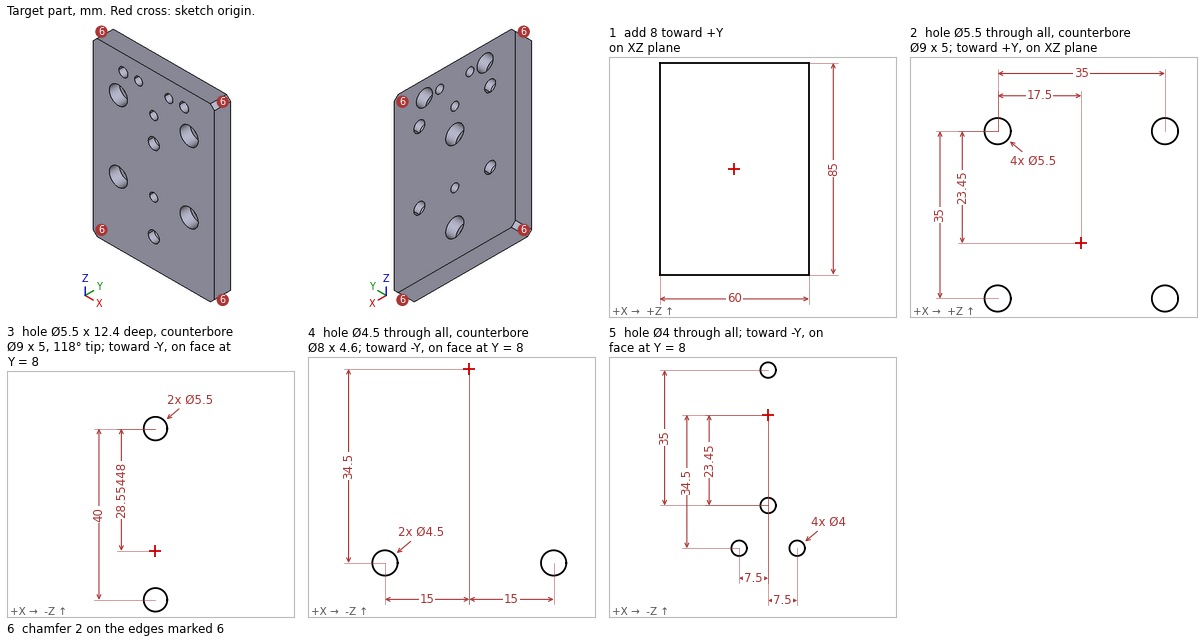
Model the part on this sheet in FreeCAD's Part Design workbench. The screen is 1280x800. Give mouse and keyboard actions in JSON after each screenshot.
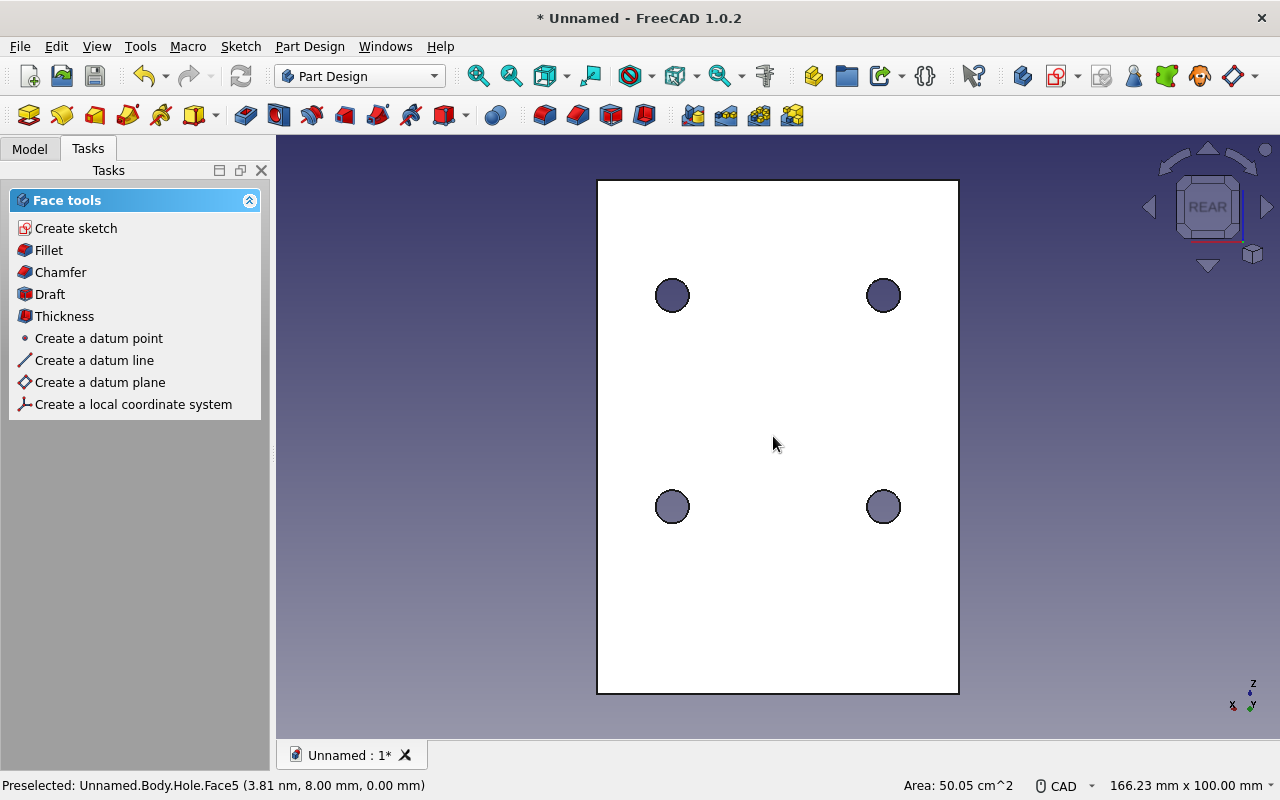
{"action": "left_click", "coordinate": [1056, 76]}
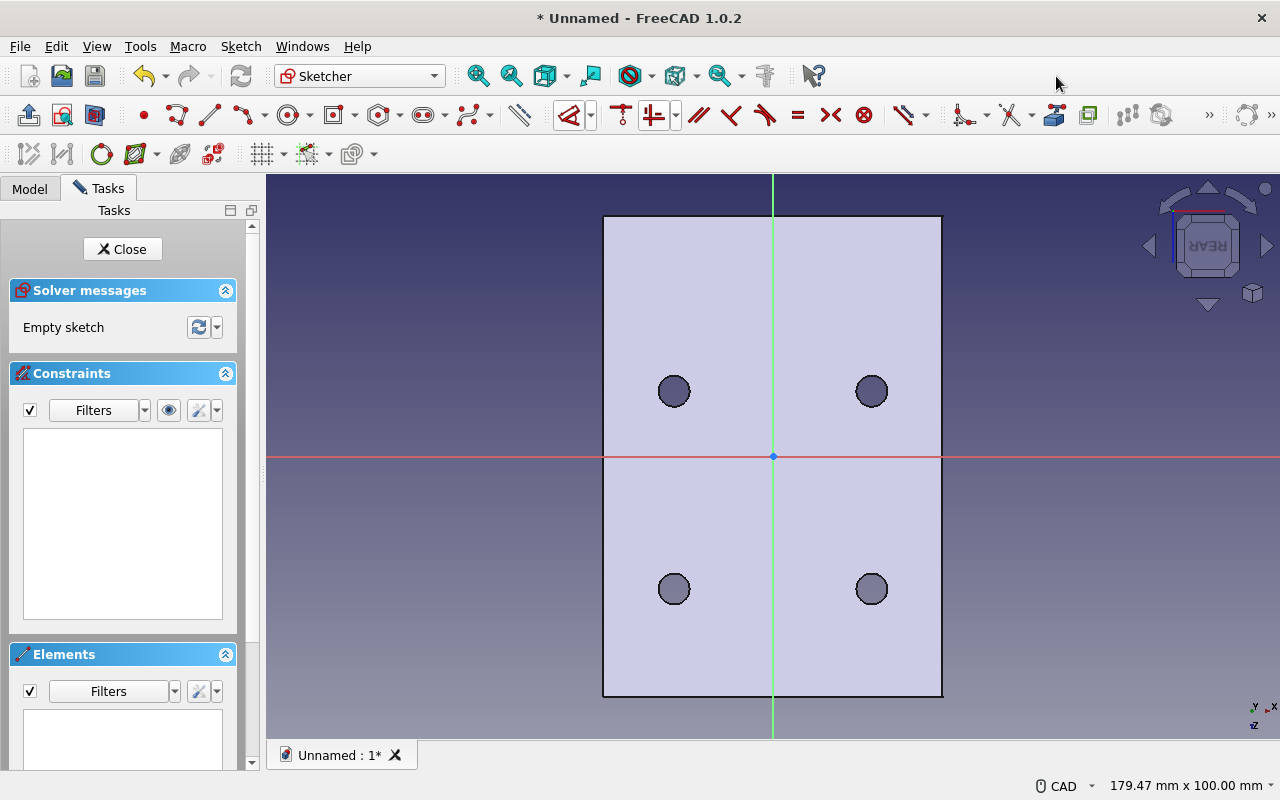
{"action": "scroll", "coordinate": [912, 310], "scroll_direction": "up", "scroll_amount": 2}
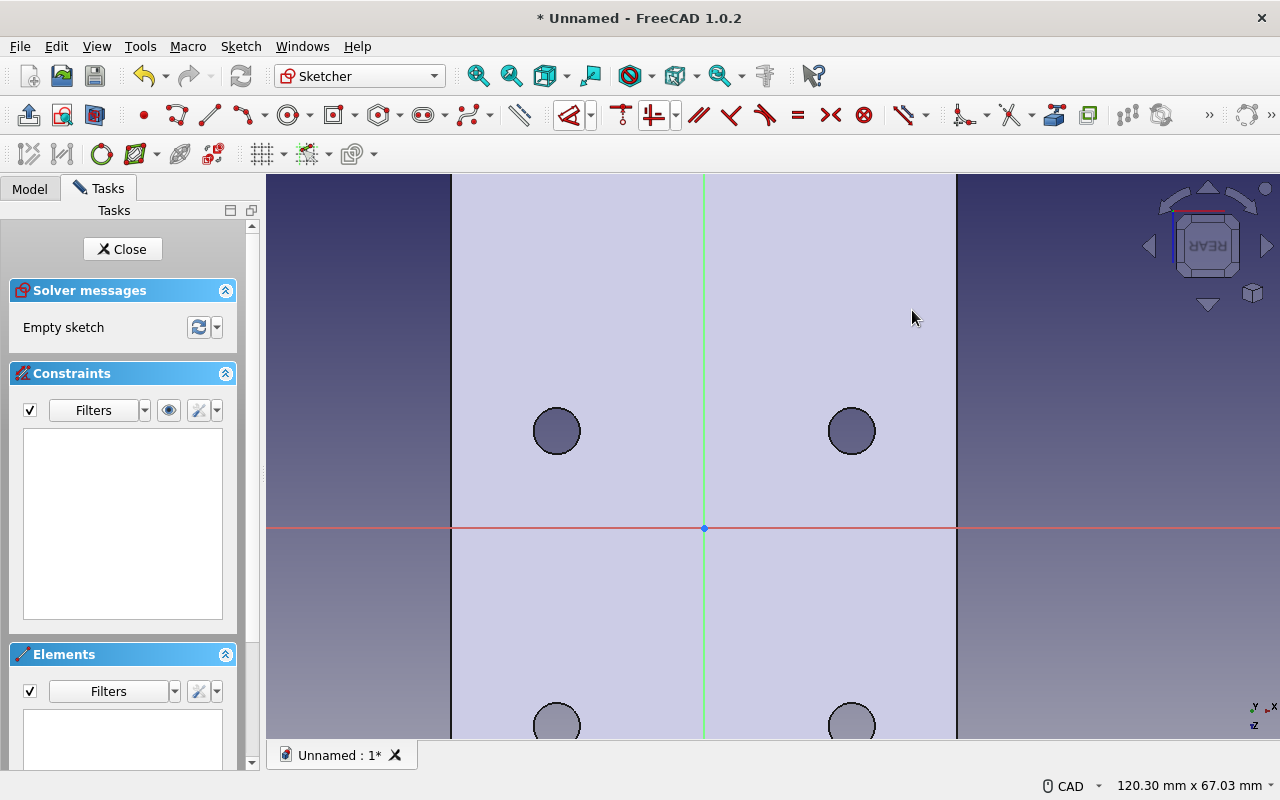
{"action": "left_click", "coordinate": [288, 116]}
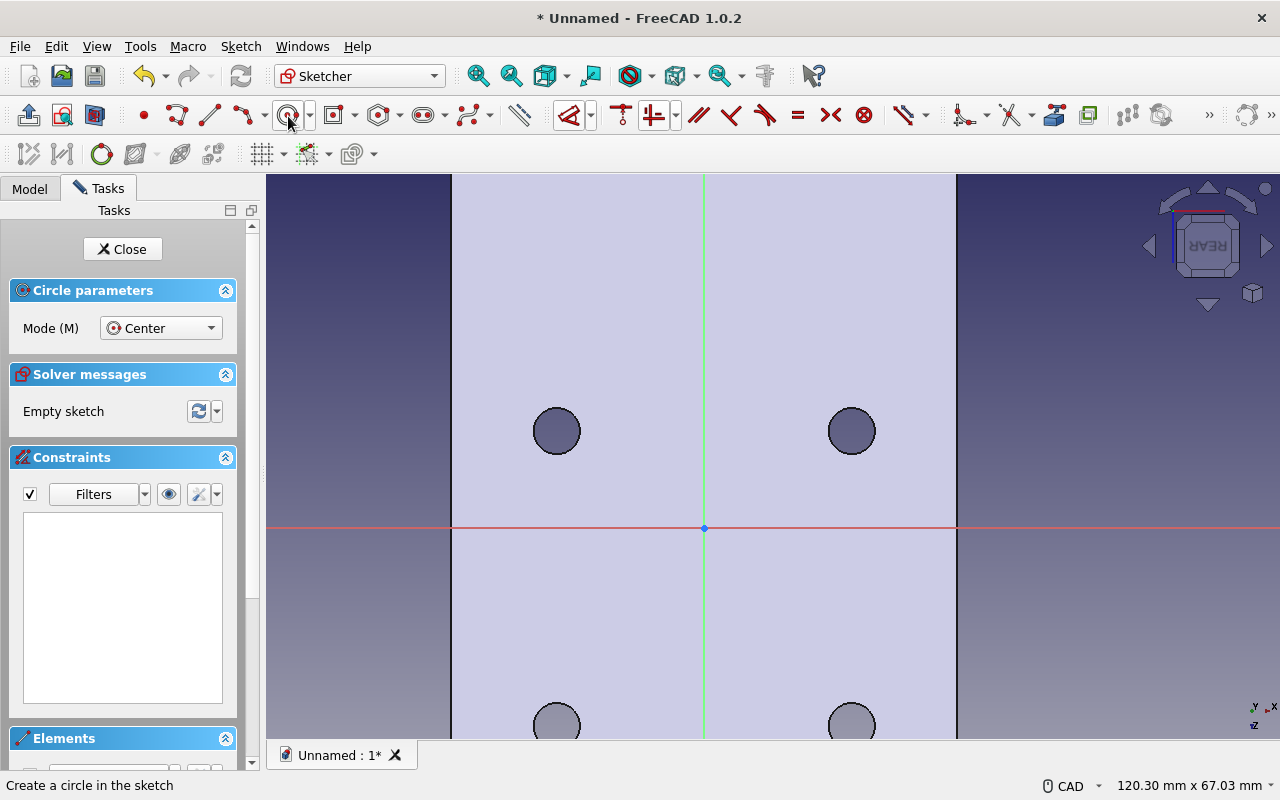
{"action": "left_click", "coordinate": [704, 288]}
{"action": "left_click", "coordinate": [721, 271]}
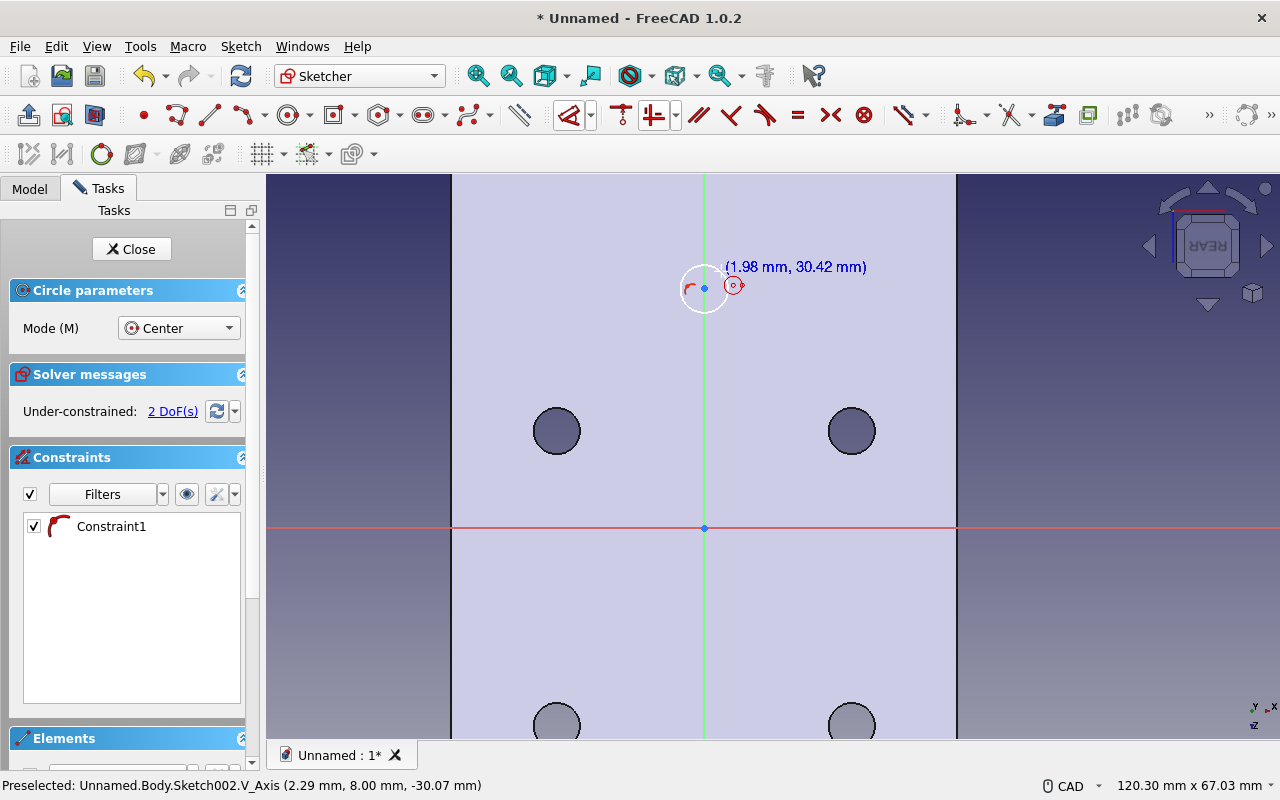
{"action": "left_click", "coordinate": [704, 625]}
{"action": "left_click", "coordinate": [721, 609]}
{"action": "key", "text": "Escape"}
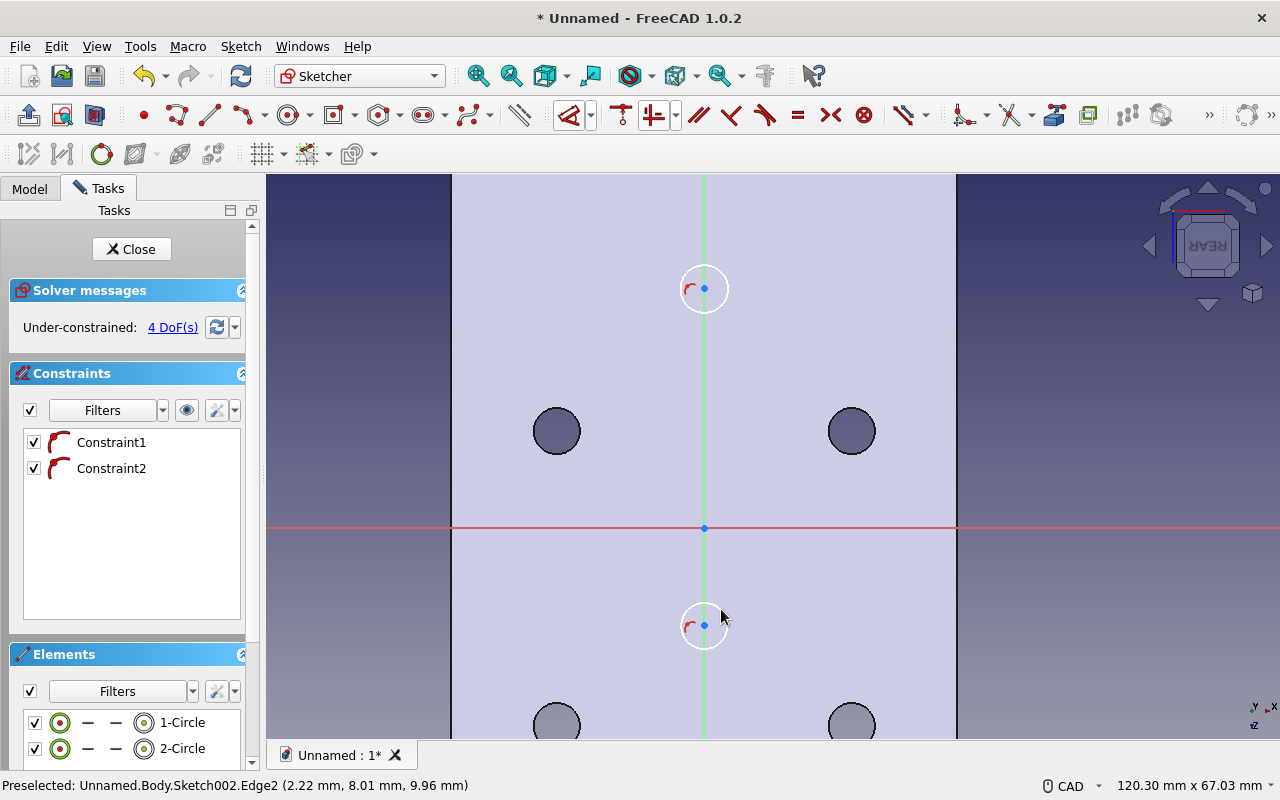
{"action": "left_click", "coordinate": [721, 272]}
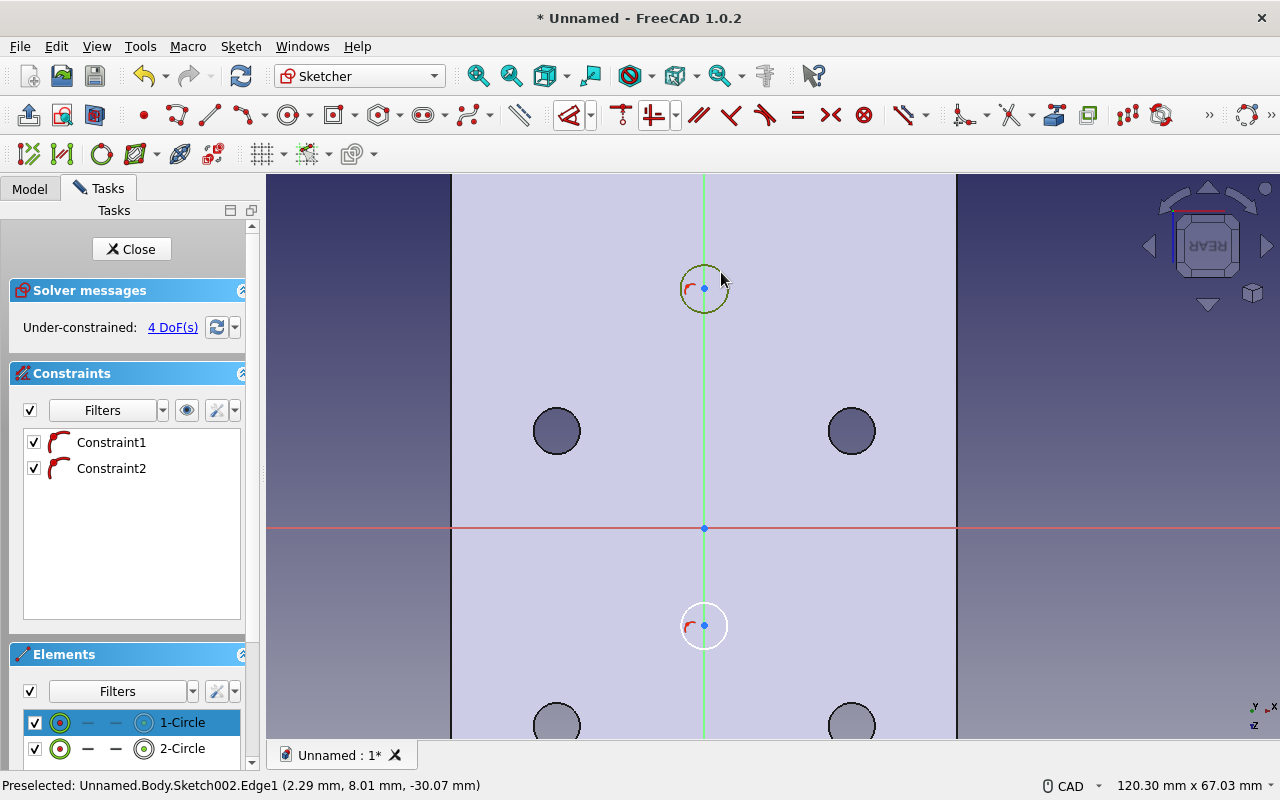
{"action": "left_click", "coordinate": [721, 610]}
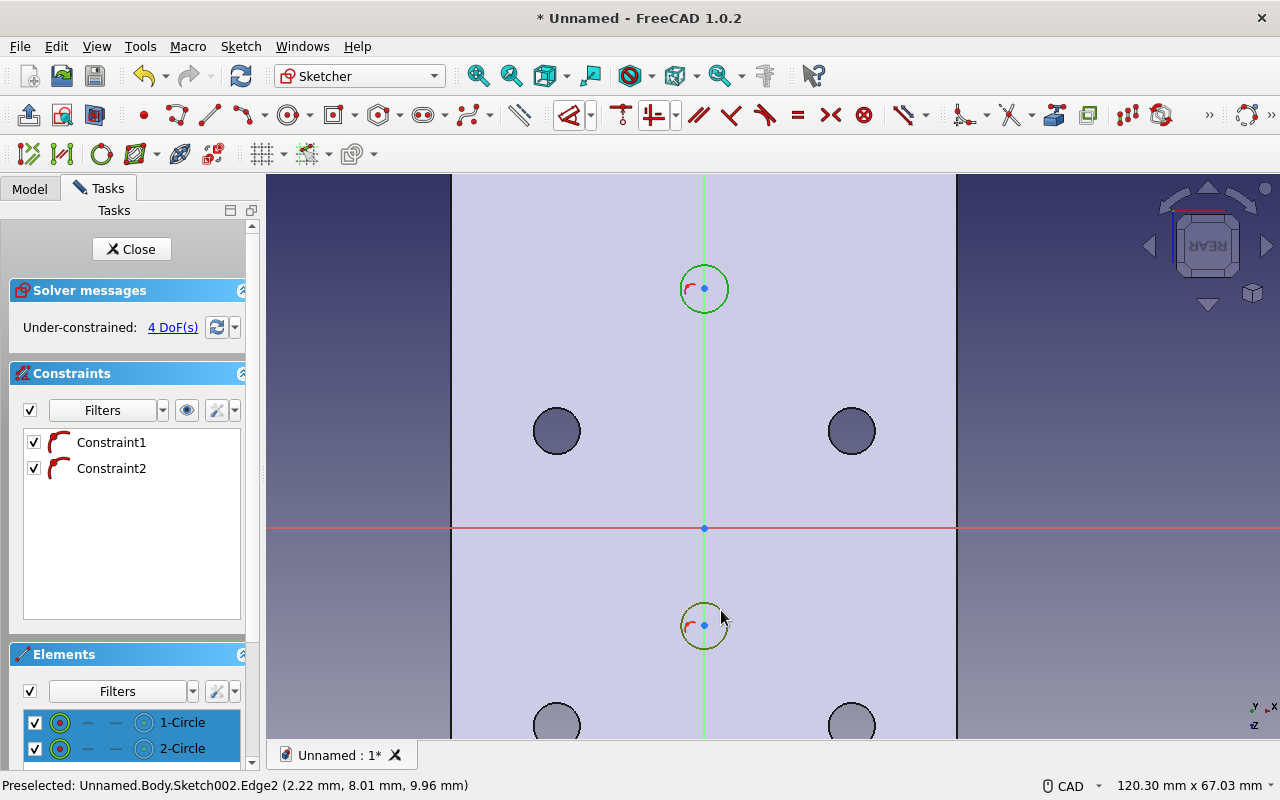
{"action": "left_click", "coordinate": [798, 116]}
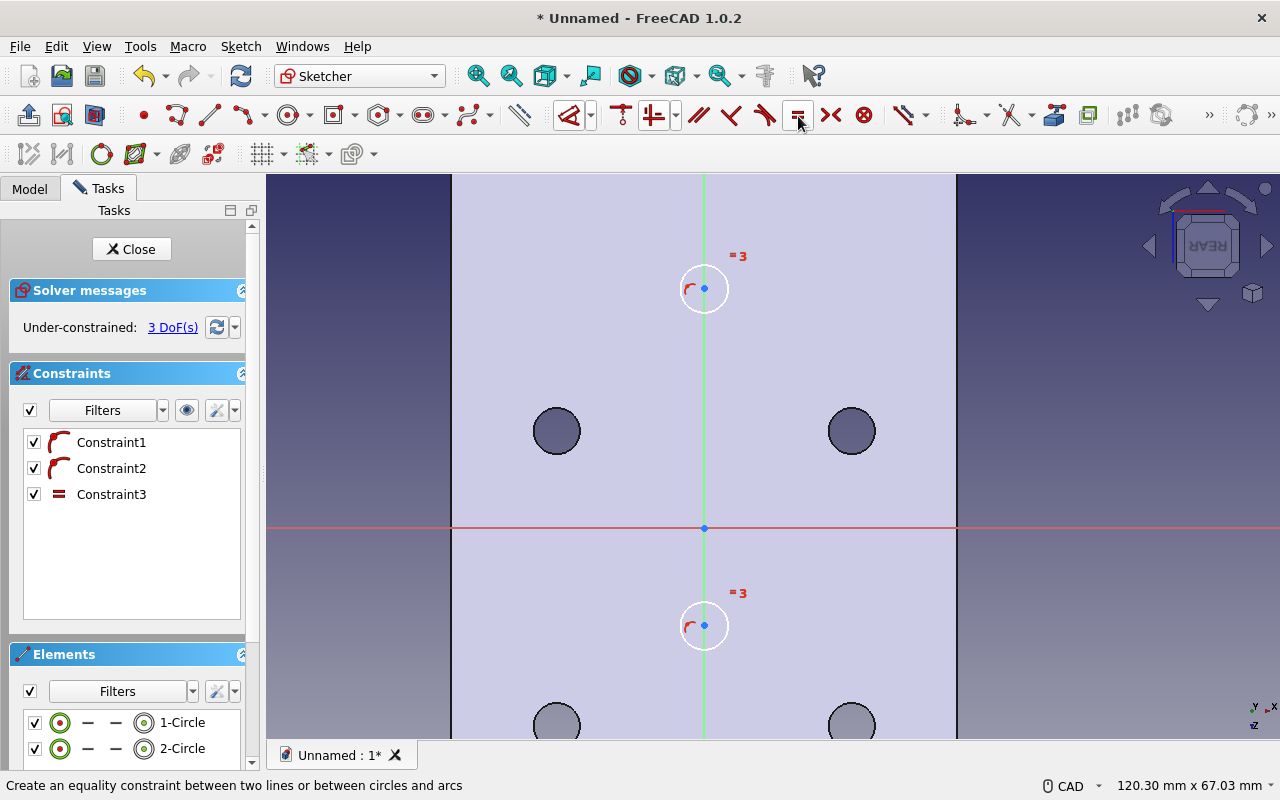
{"action": "left_click", "coordinate": [721, 272]}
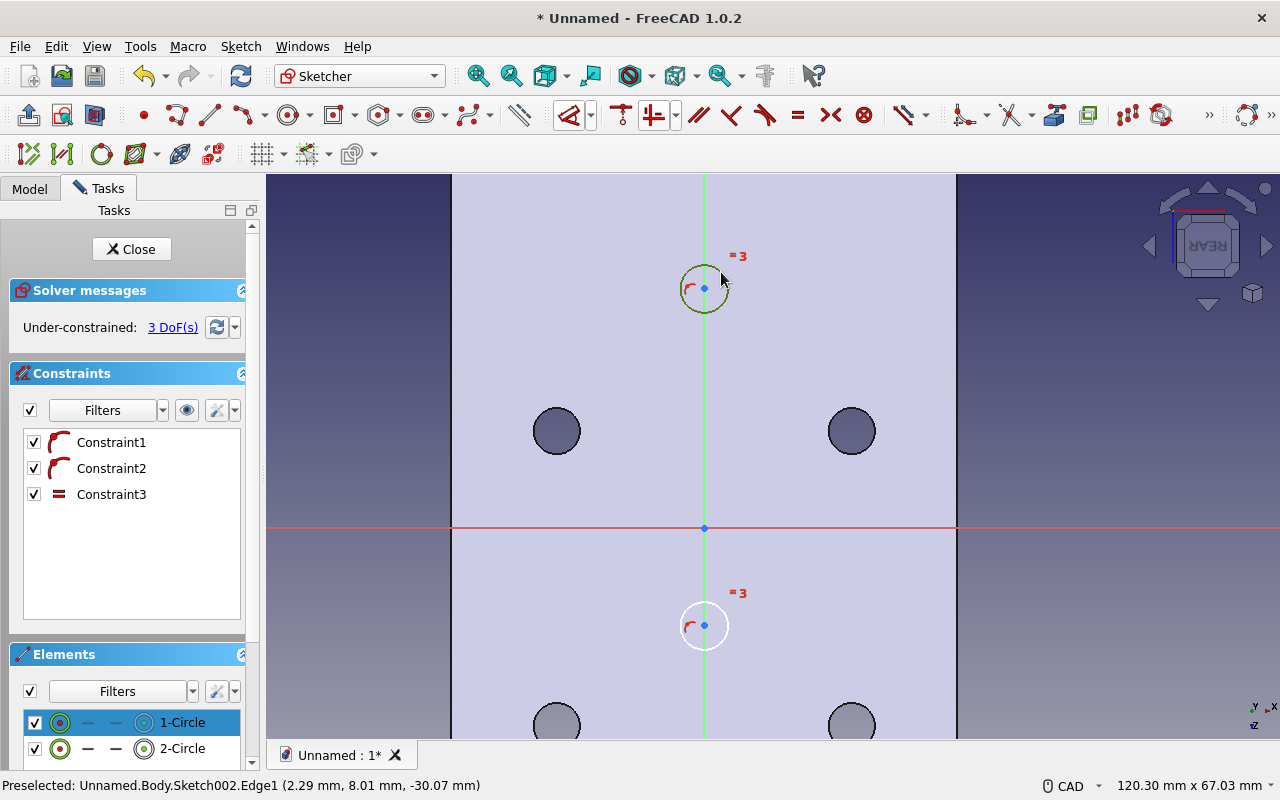
{"action": "key", "text": "k o"}